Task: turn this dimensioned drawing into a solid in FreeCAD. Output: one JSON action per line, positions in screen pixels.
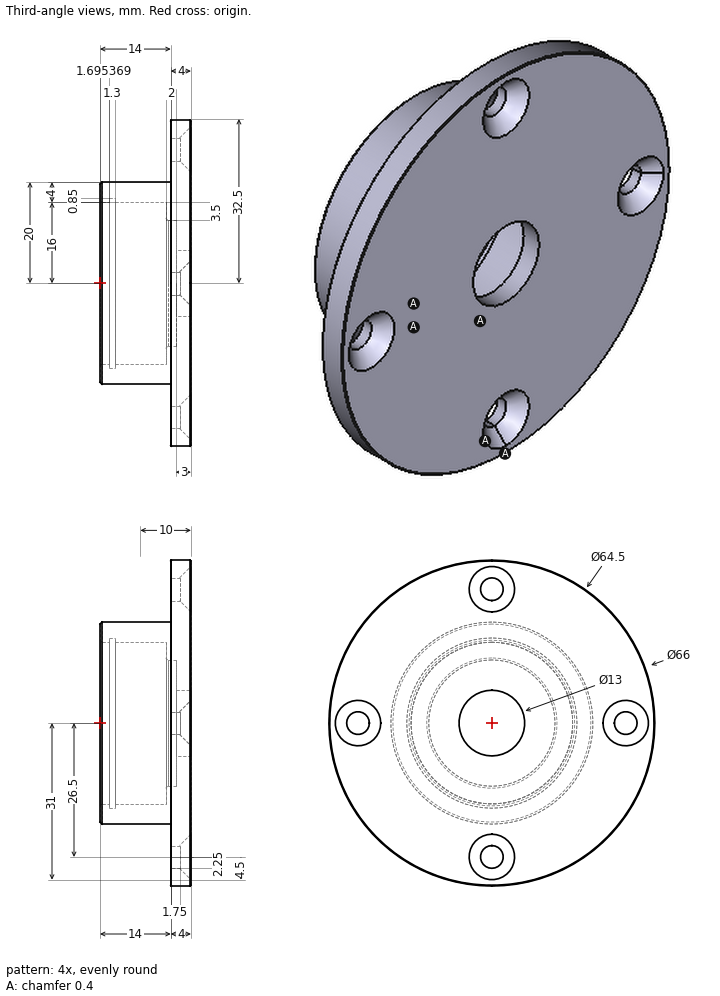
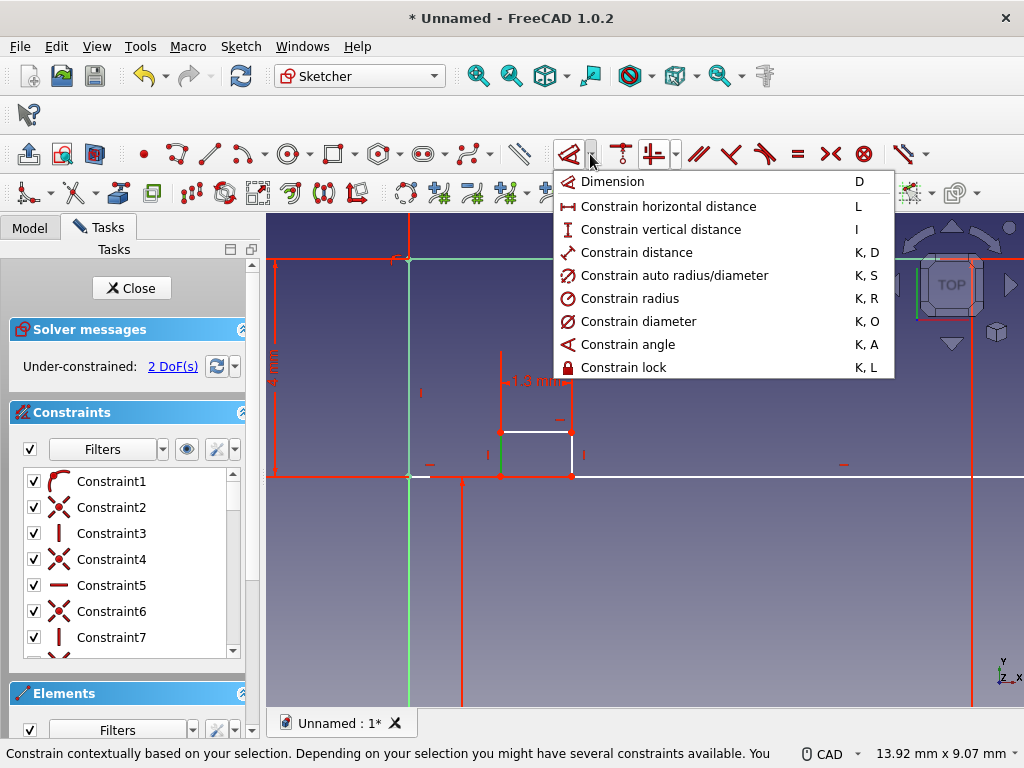
{"action": "left_click", "coordinate": [724, 230]}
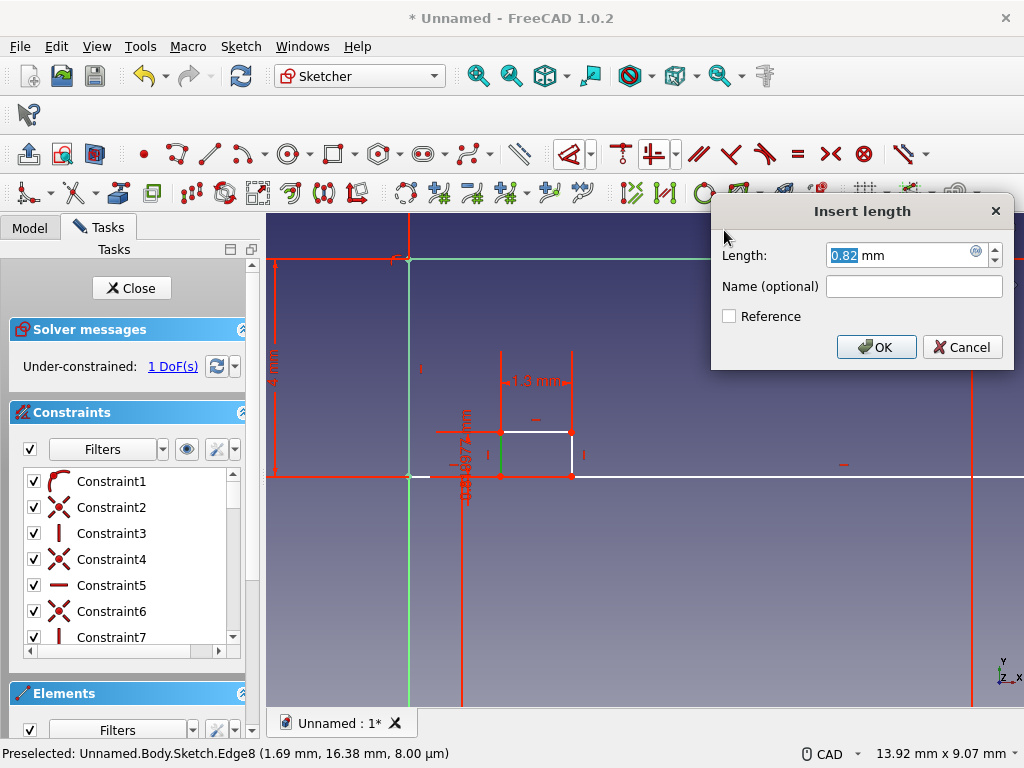
{"action": "type", "text": "0.85"}
{"action": "key", "text": "Return"}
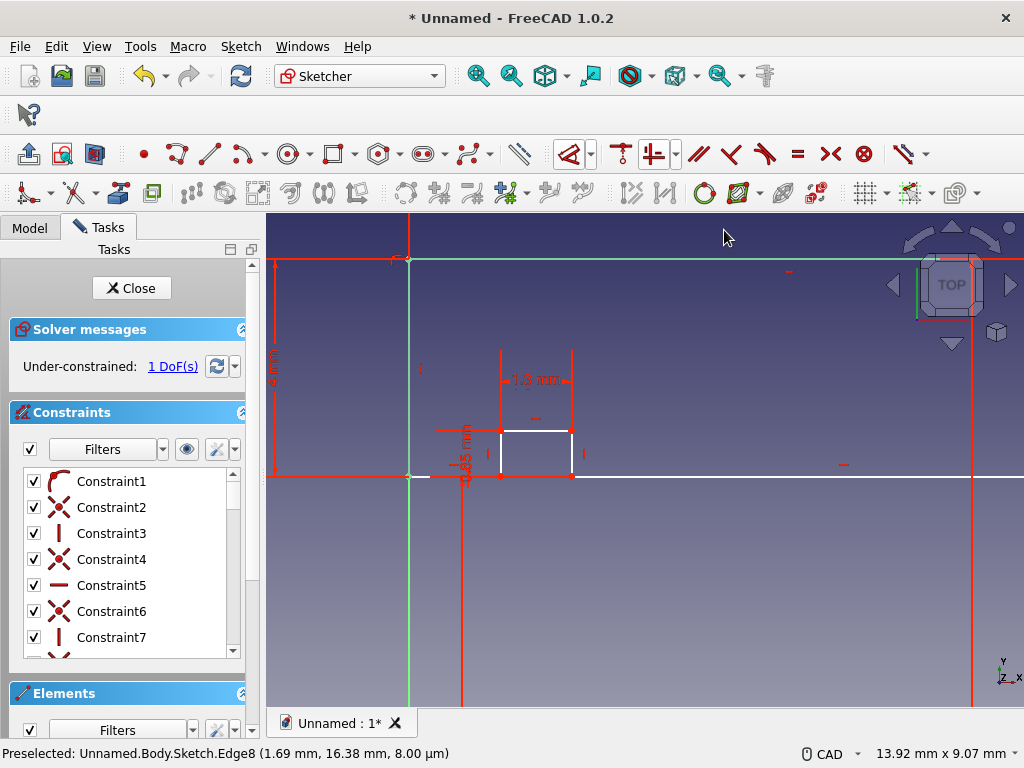
{"action": "left_click", "coordinate": [436, 477]}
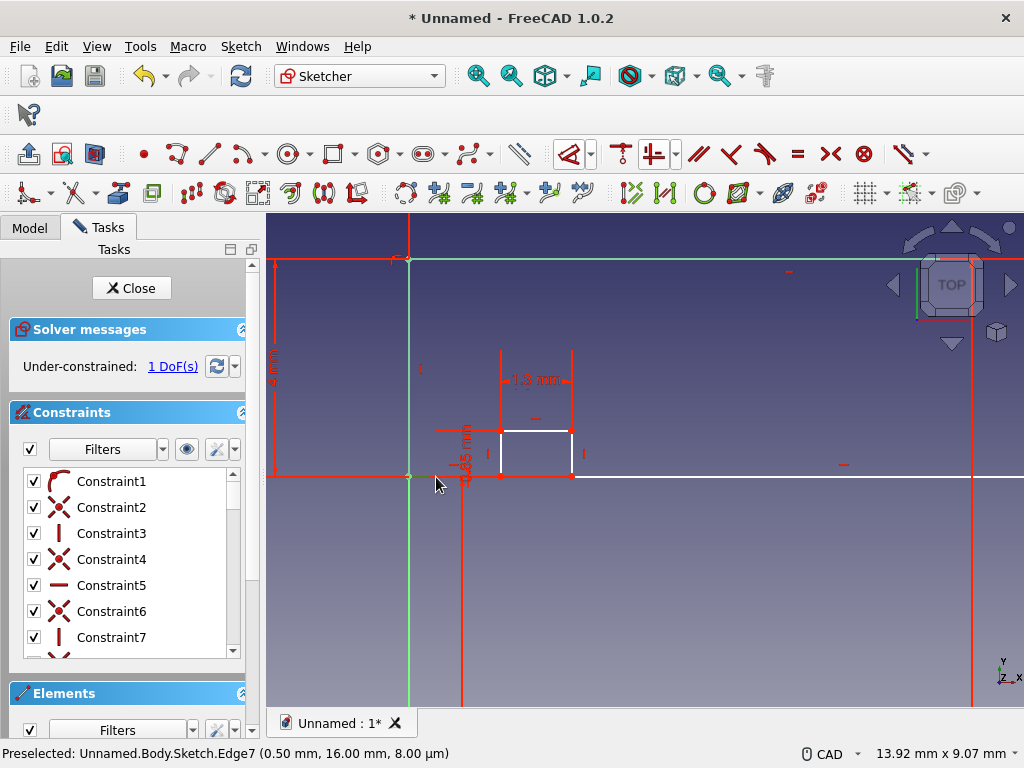
{"action": "left_click", "coordinate": [590, 154]}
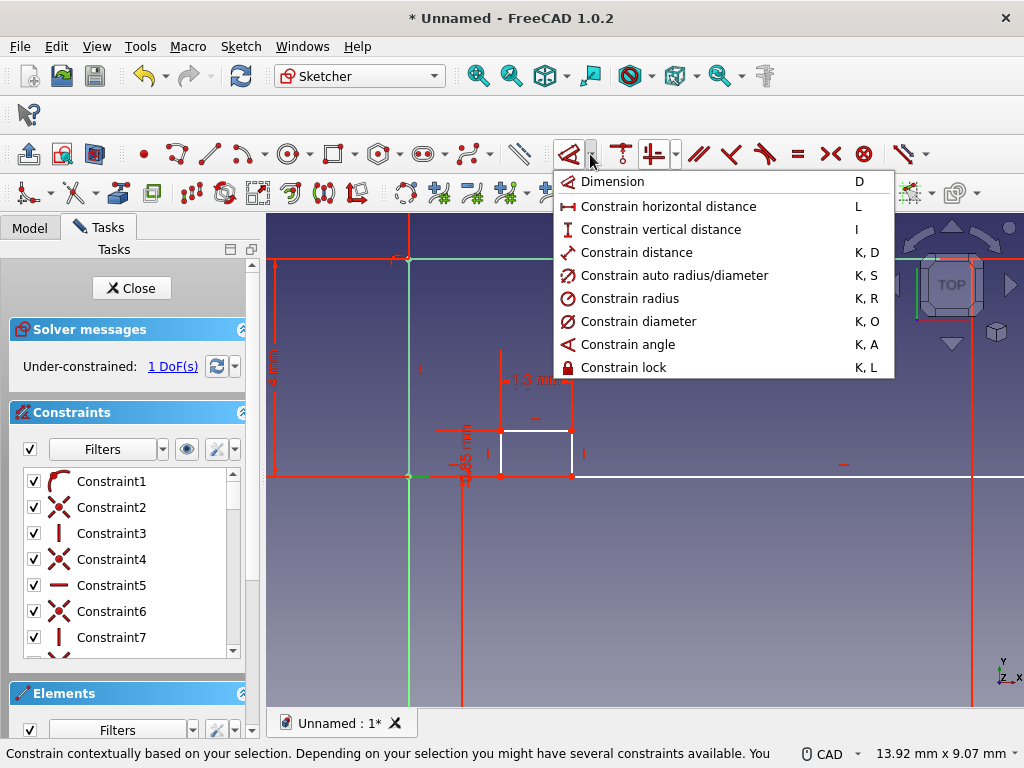
{"action": "left_click", "coordinate": [724, 206]}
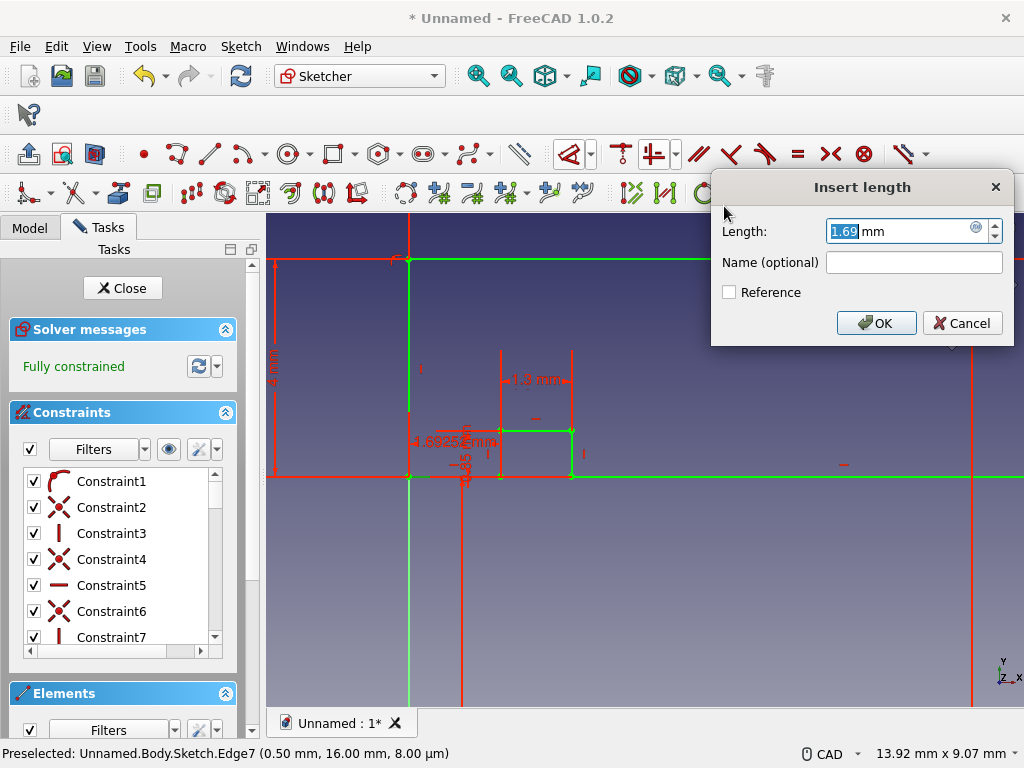
{"action": "type", "text": "1.695369"}
{"action": "key", "text": "Return"}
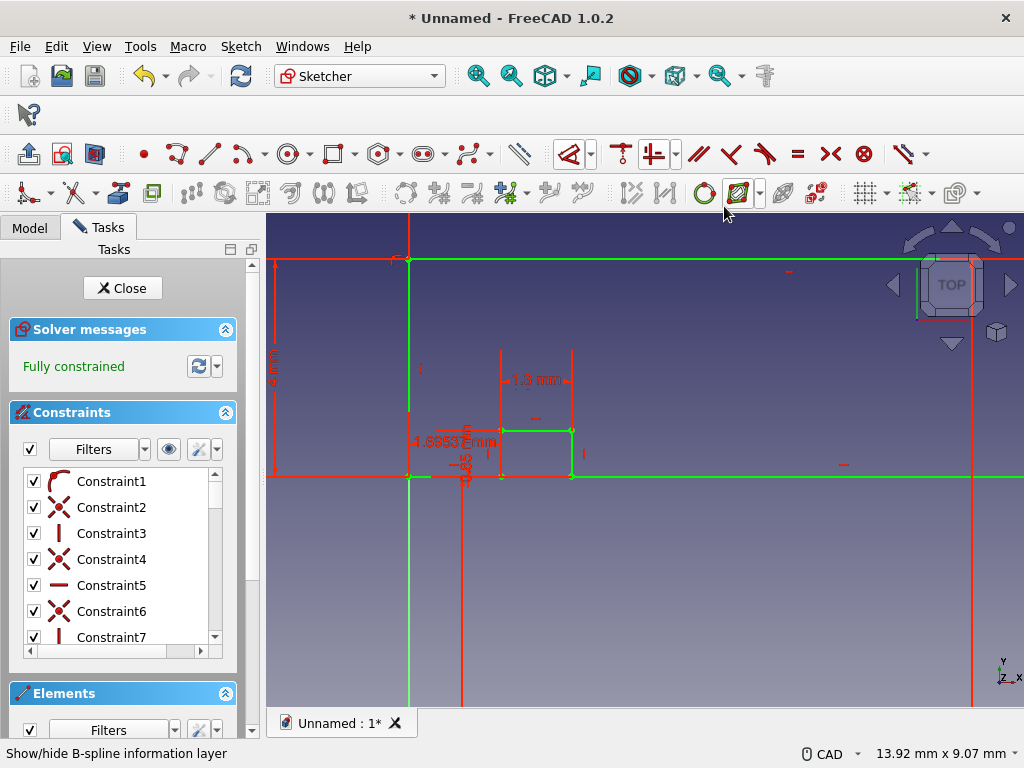
{"action": "left_click", "coordinate": [123, 288]}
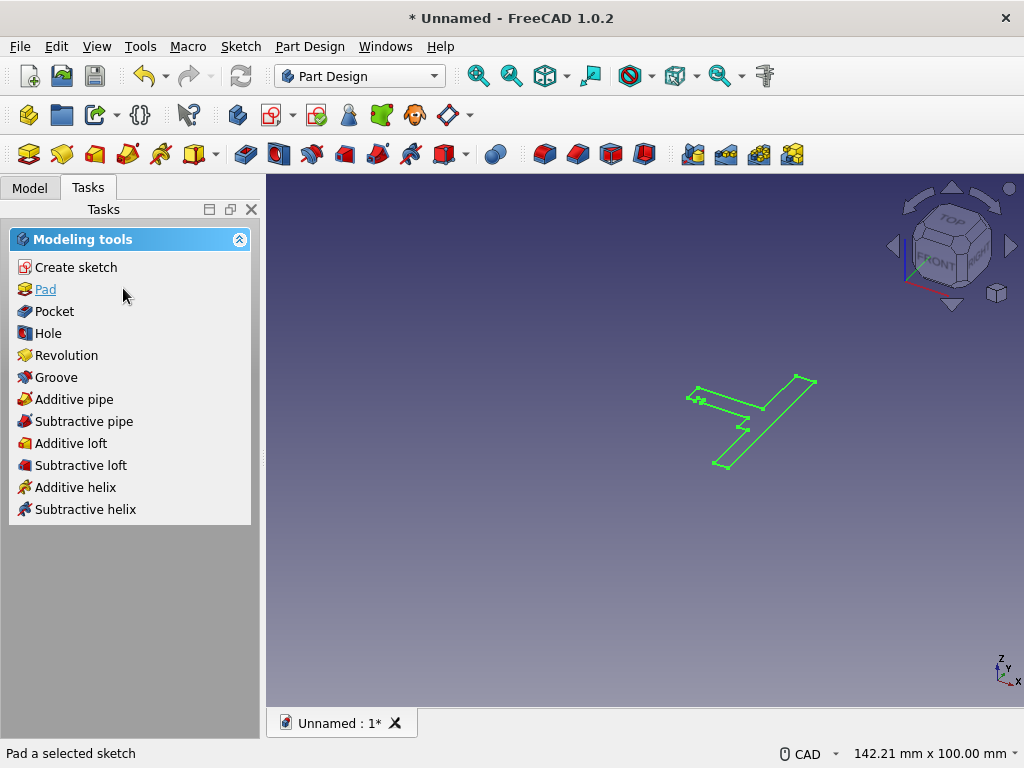
{"action": "left_click", "coordinate": [62, 154]}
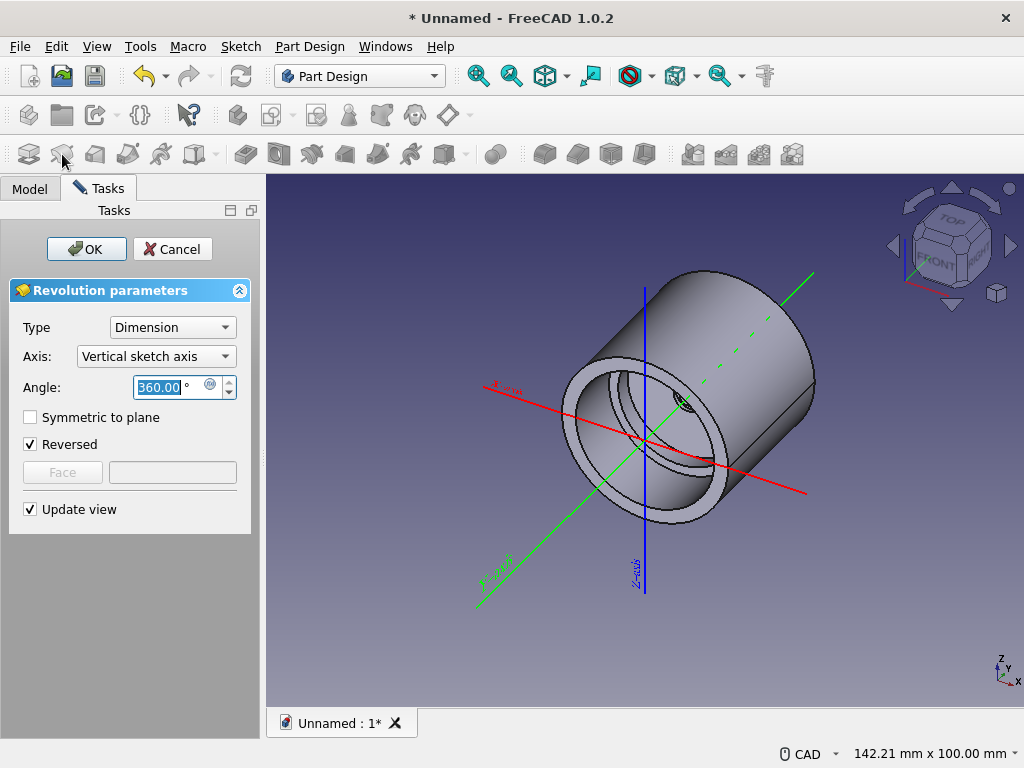
{"action": "left_click", "coordinate": [157, 356]}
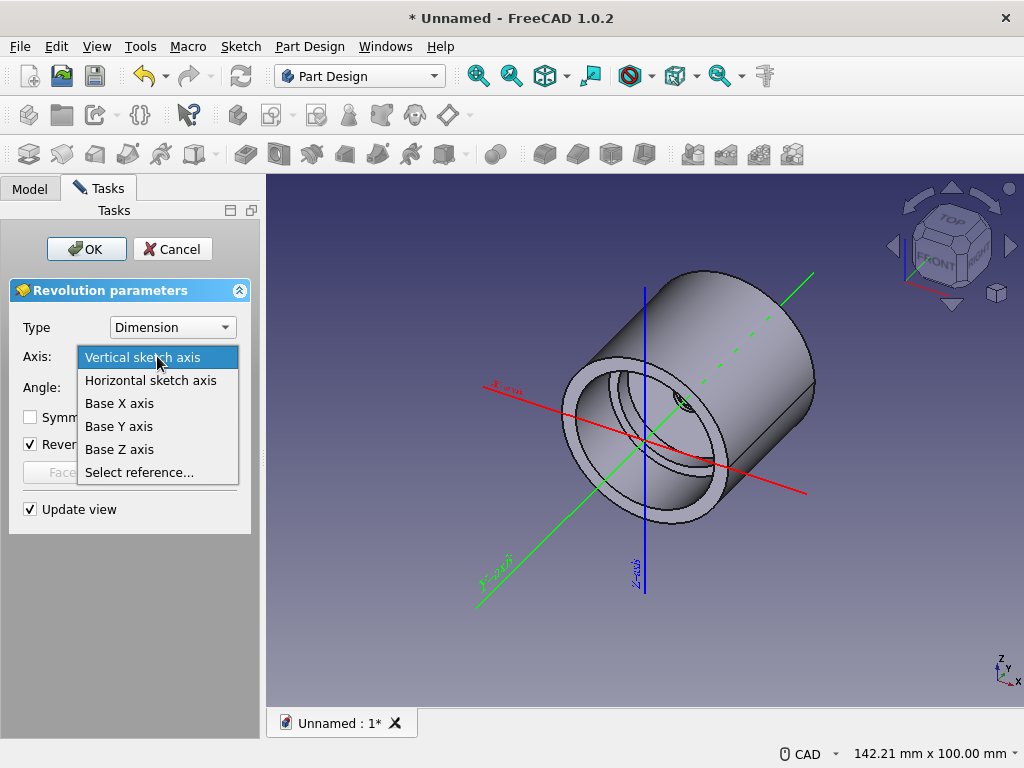
{"action": "left_click", "coordinate": [156, 380]}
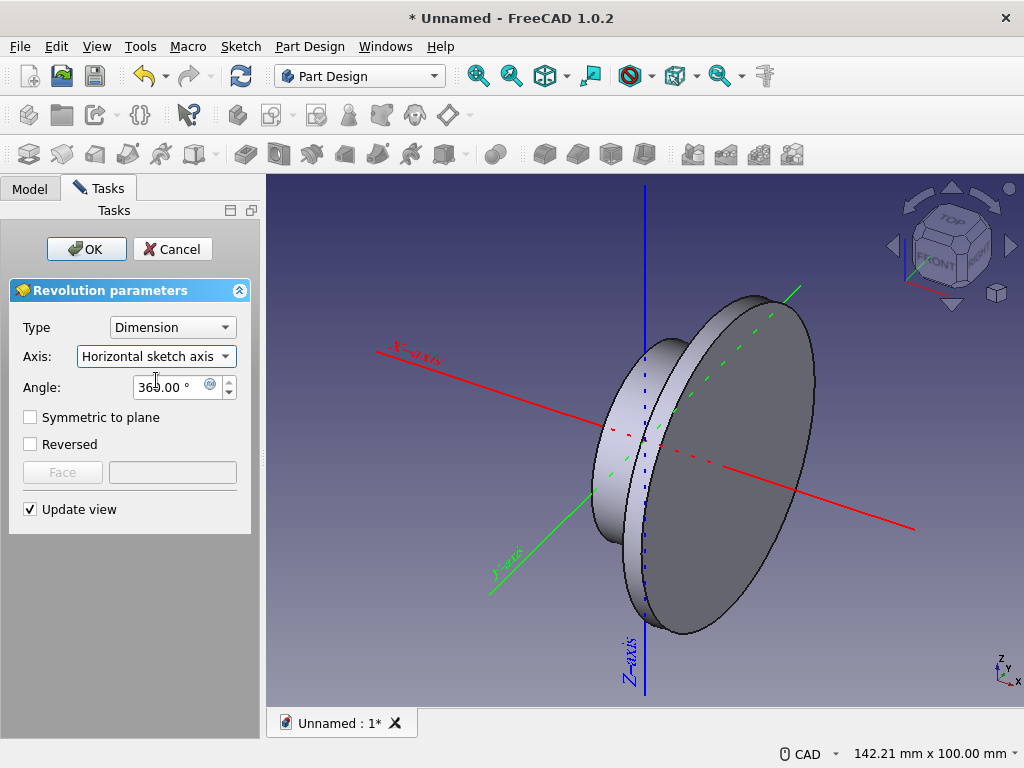
{"action": "left_click", "coordinate": [87, 249]}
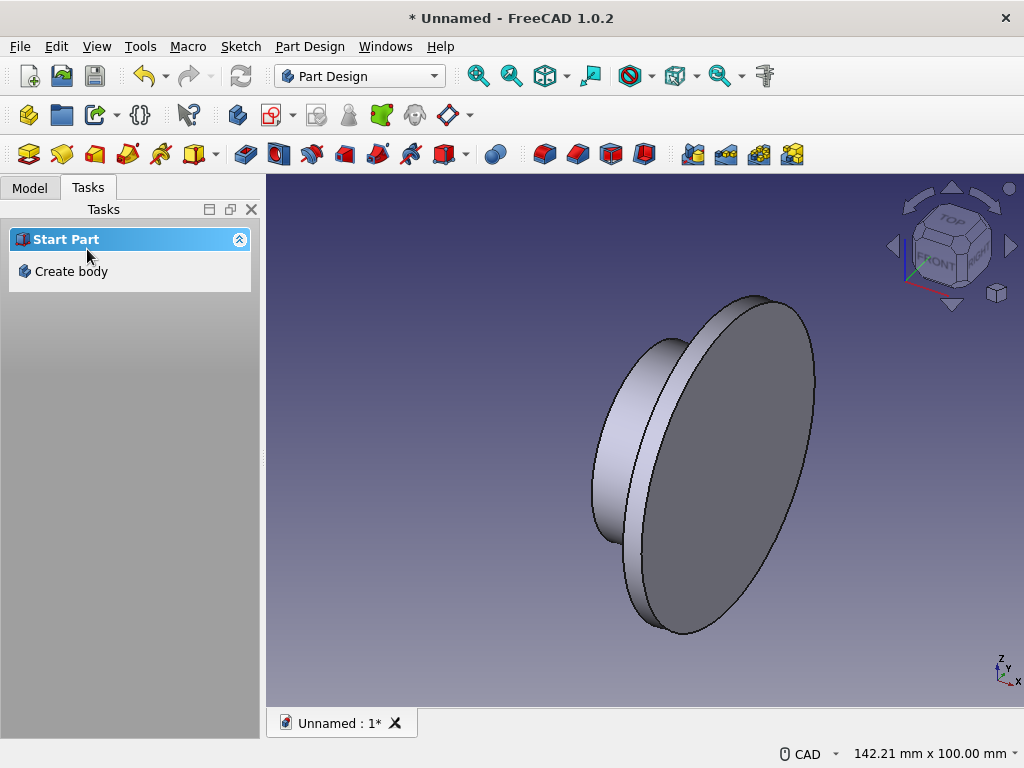
{"action": "left_click", "coordinate": [270, 116]}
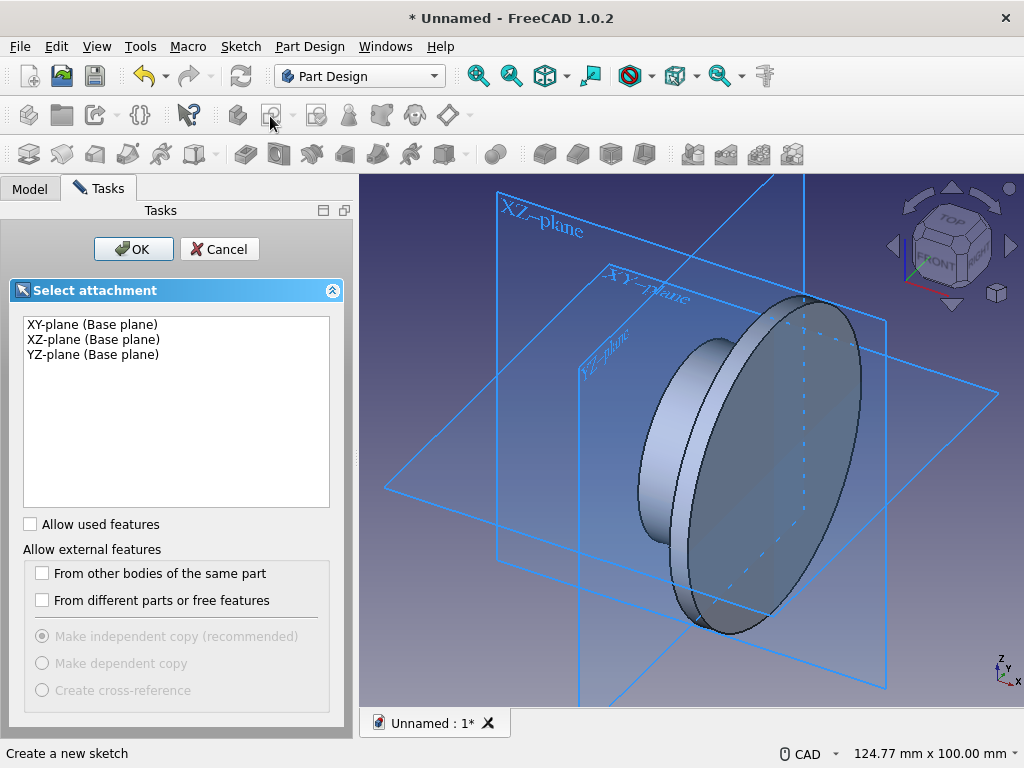
{"action": "left_click", "coordinate": [84, 340]}